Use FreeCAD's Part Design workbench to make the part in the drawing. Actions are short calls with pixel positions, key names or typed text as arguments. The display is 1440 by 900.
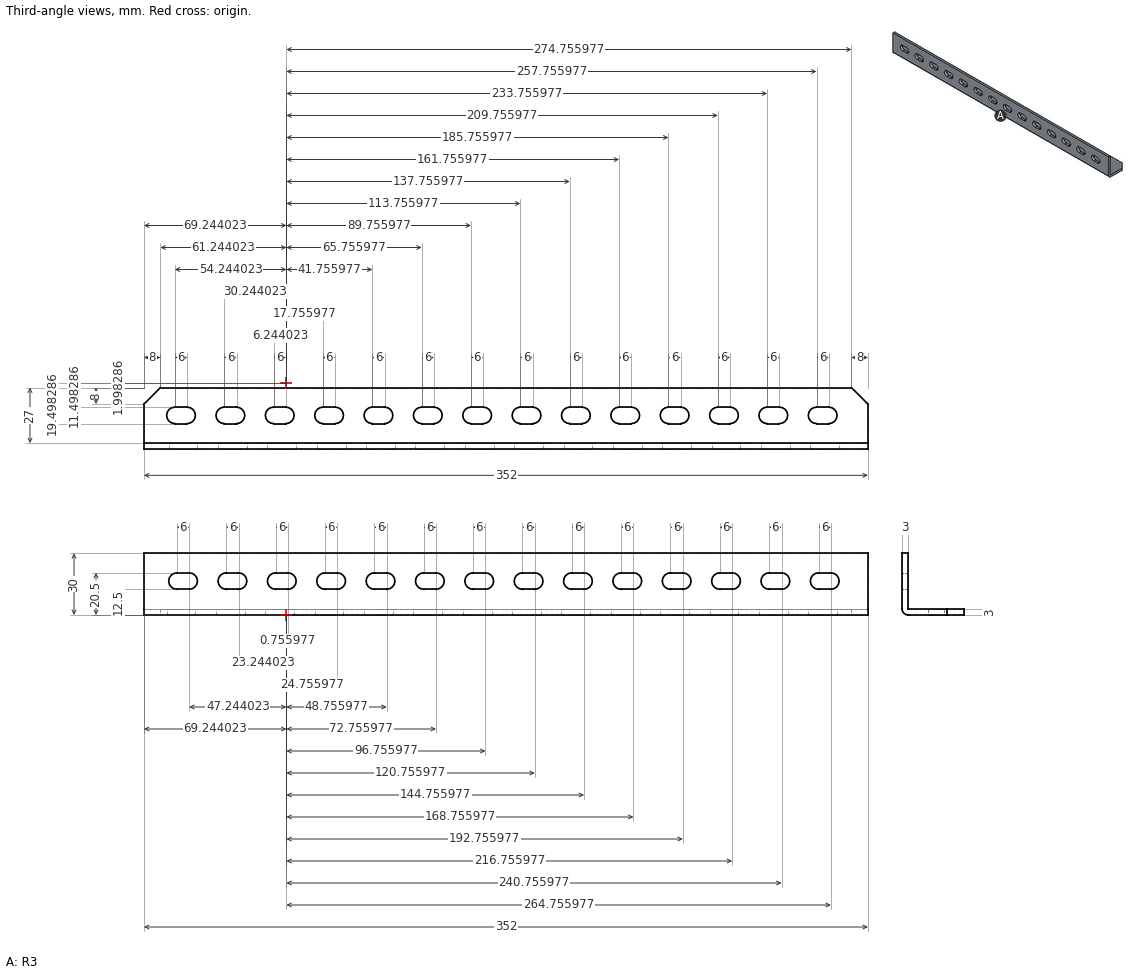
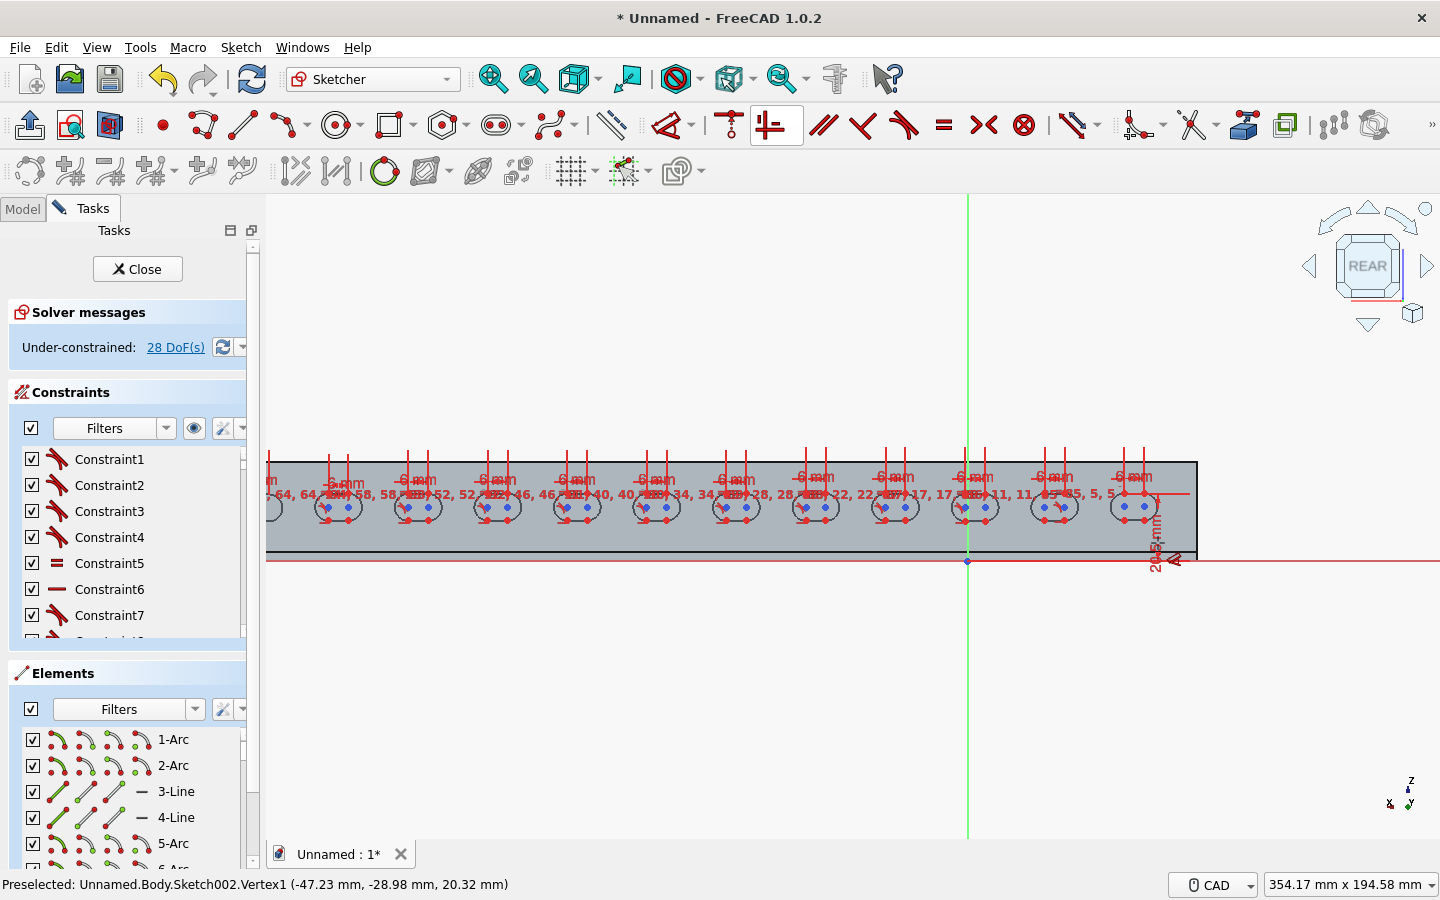
click(1124, 520)
click(934, 541)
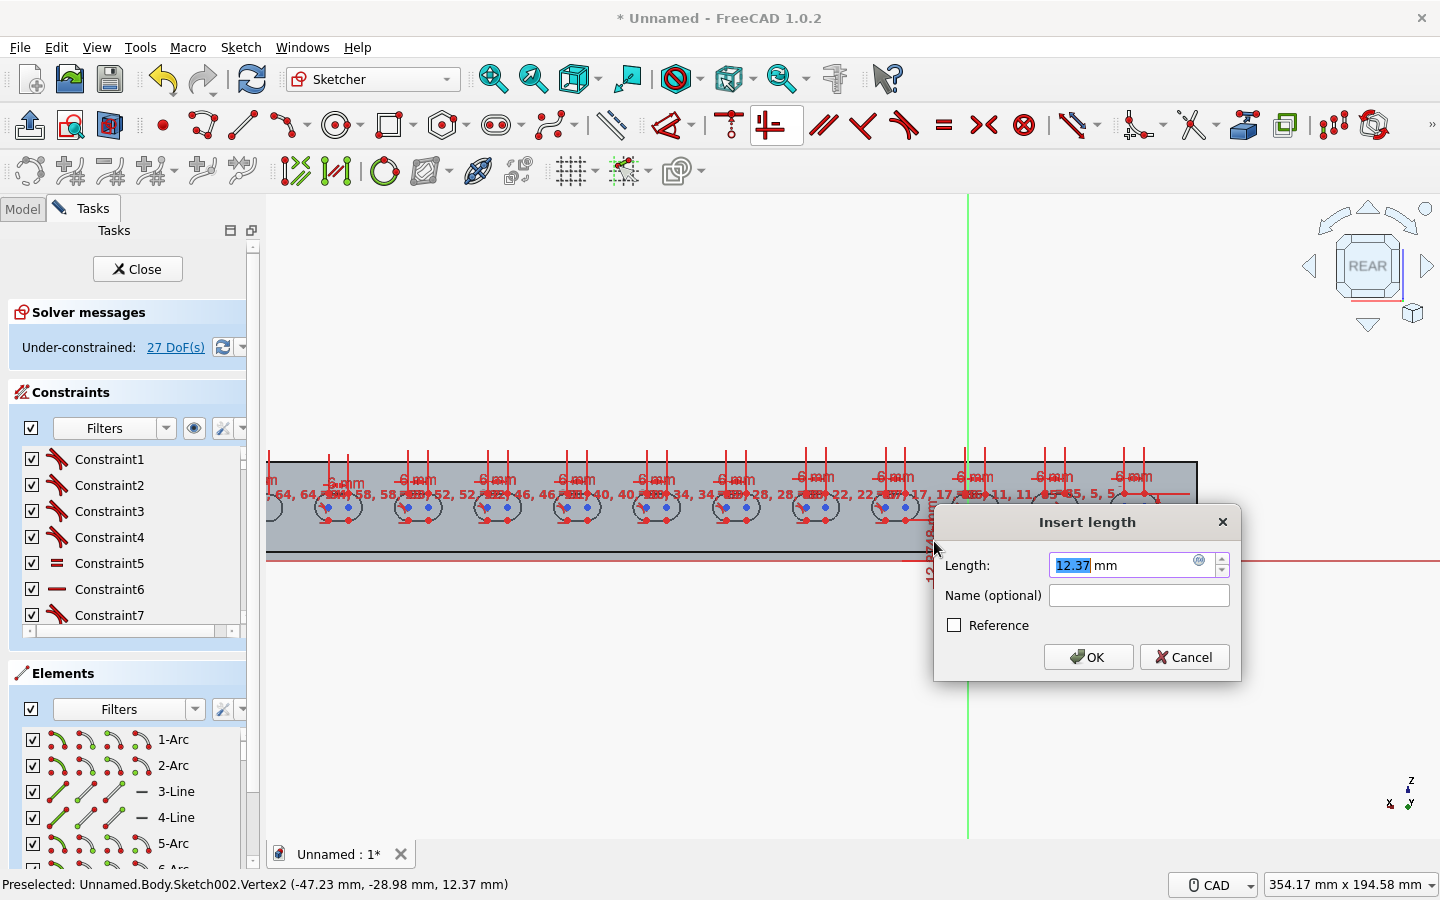
text(12.5)
key(Return)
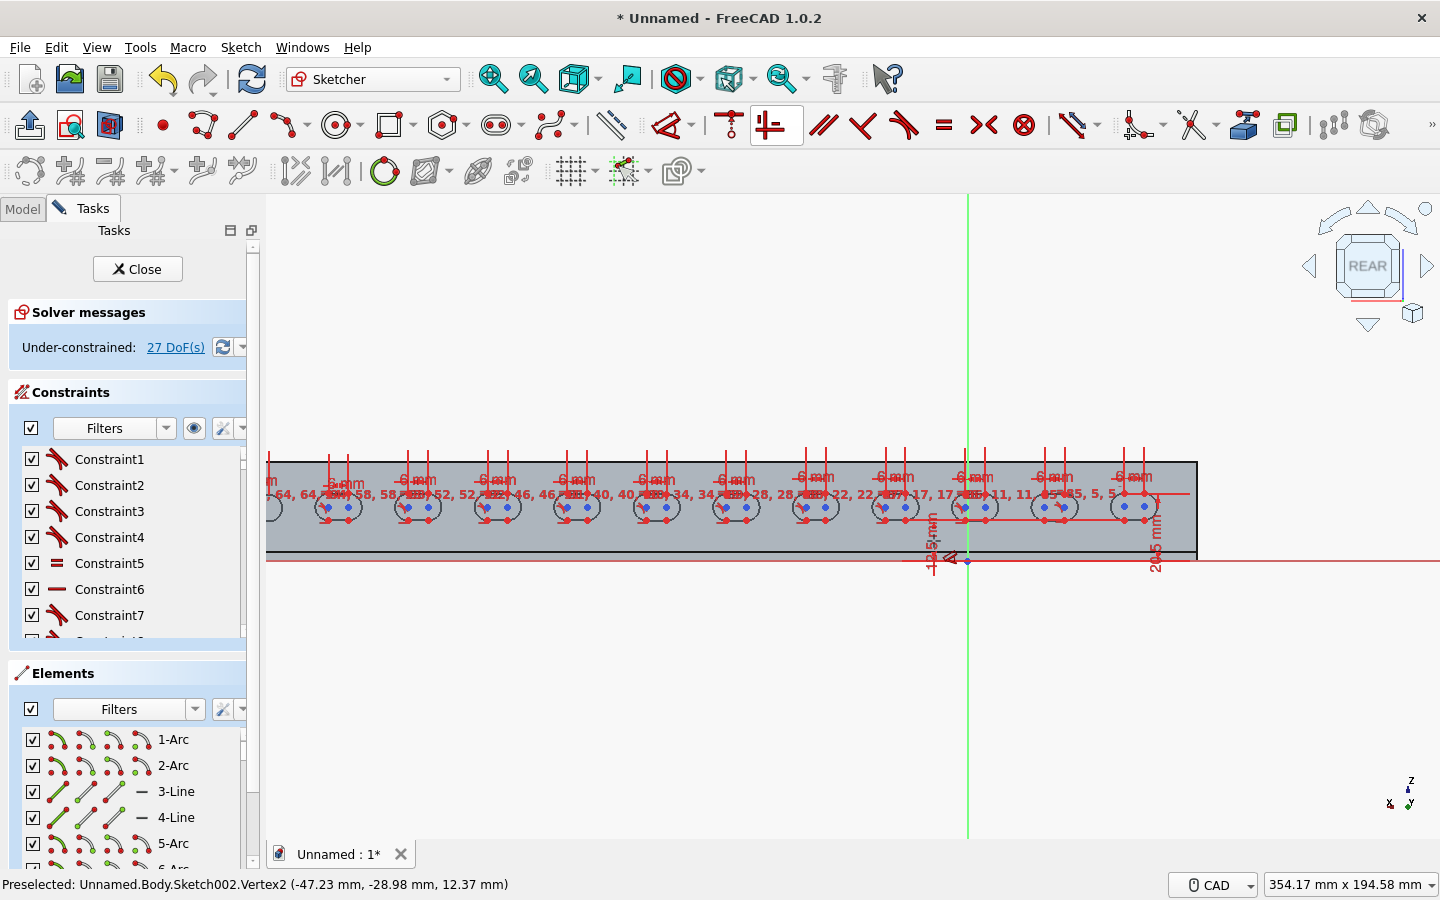
click(1045, 494)
click(1079, 543)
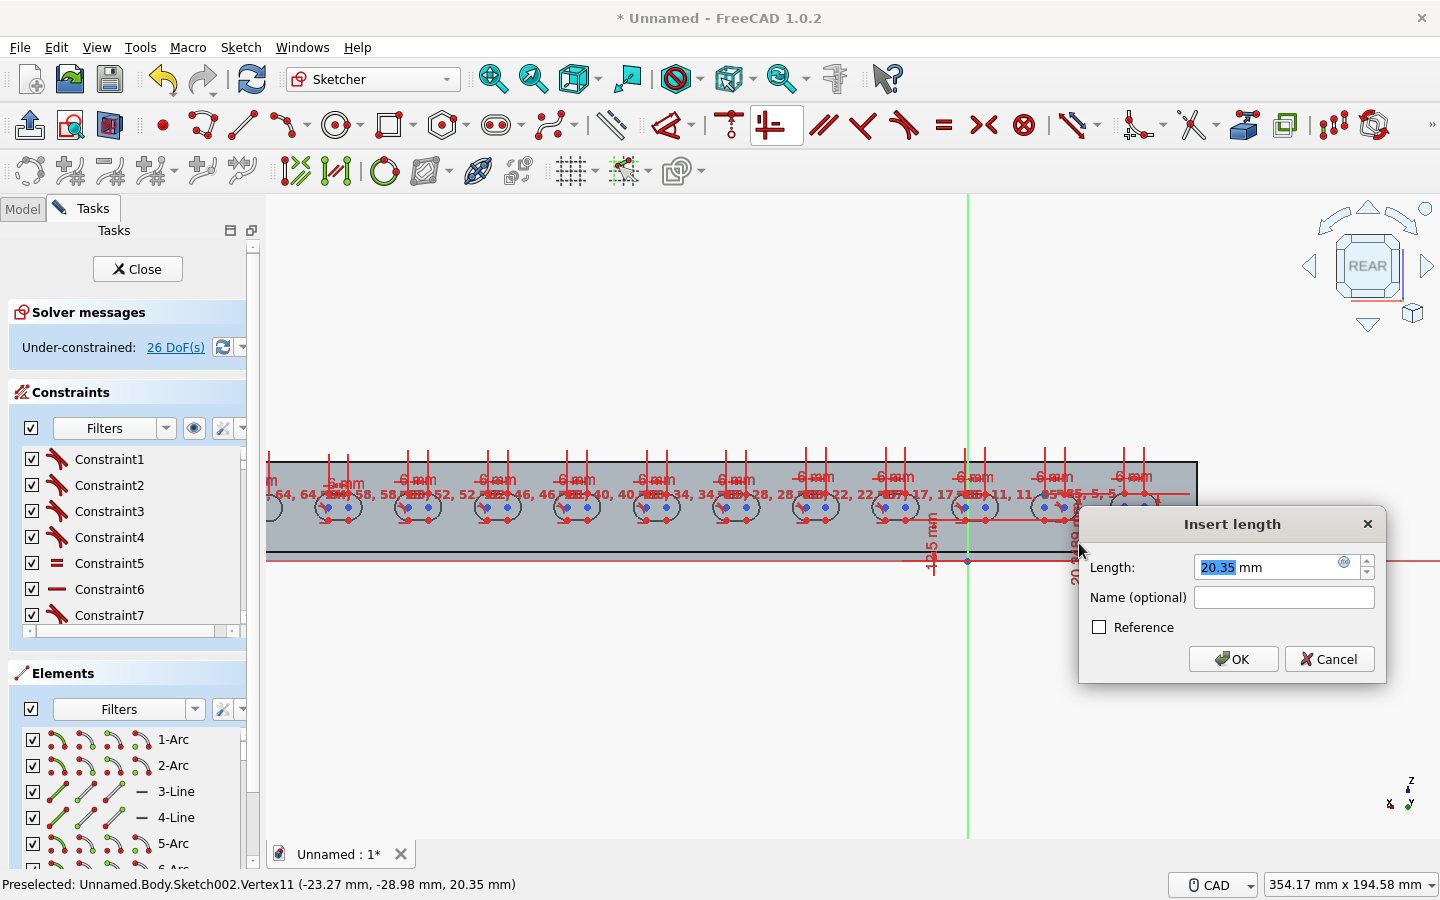
text(20.5)
key(Return)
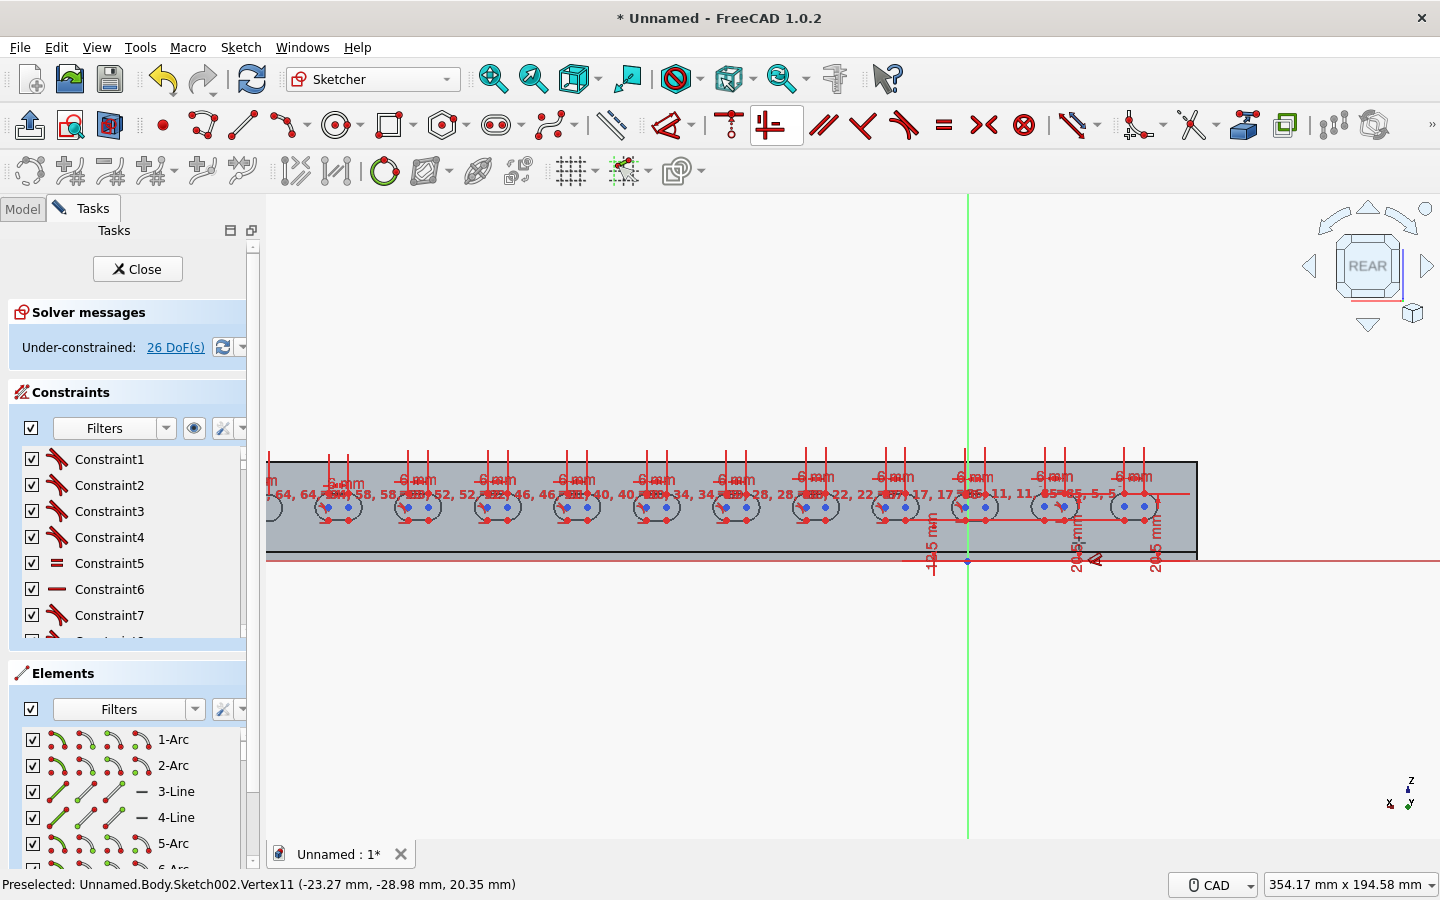
click(965, 494)
click(931, 512)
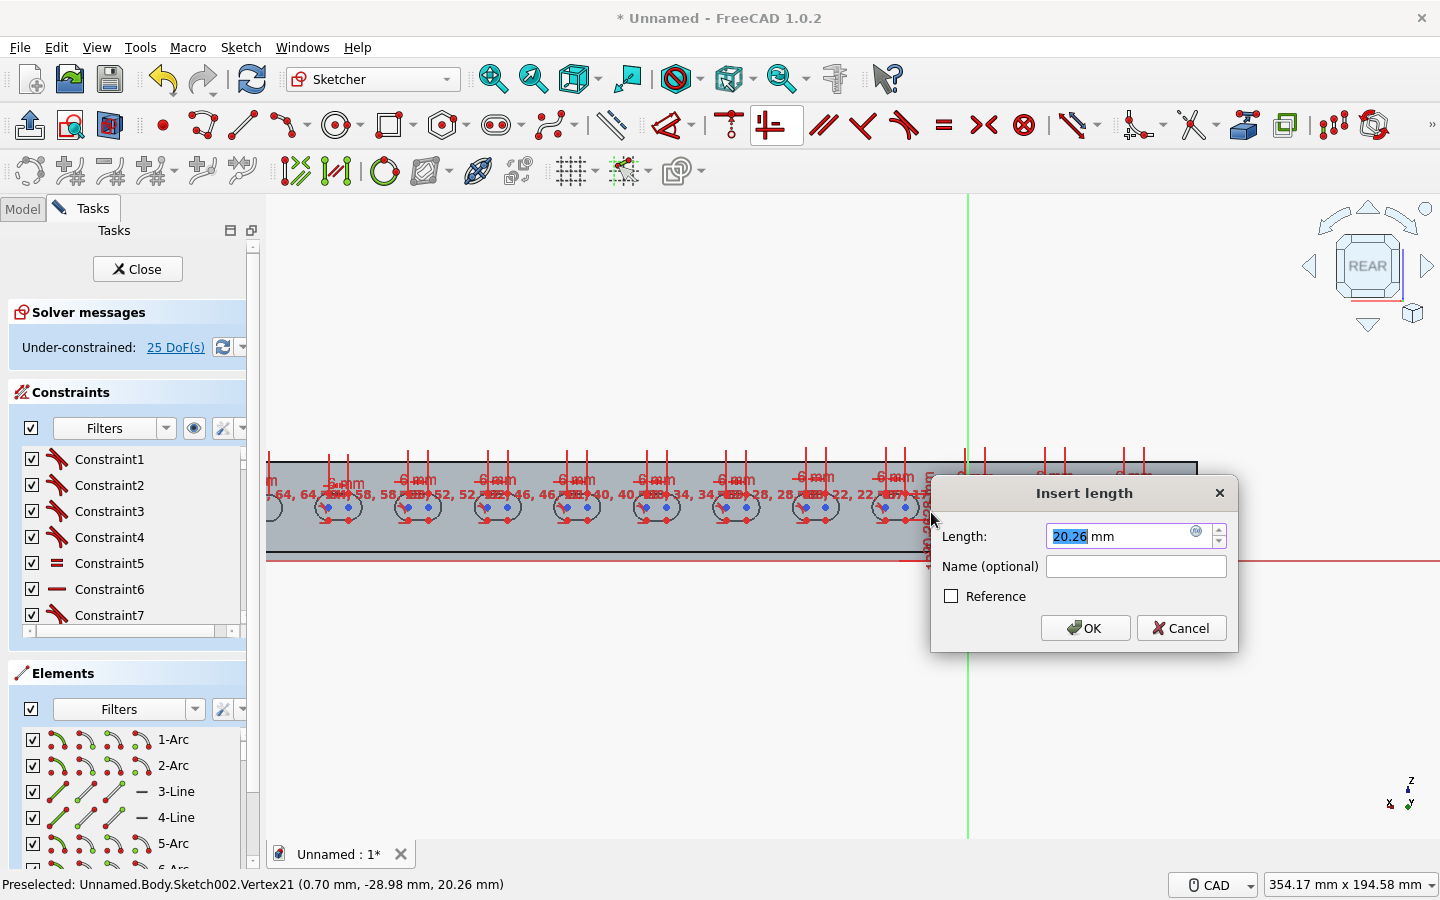
text(20.5)
key(Return)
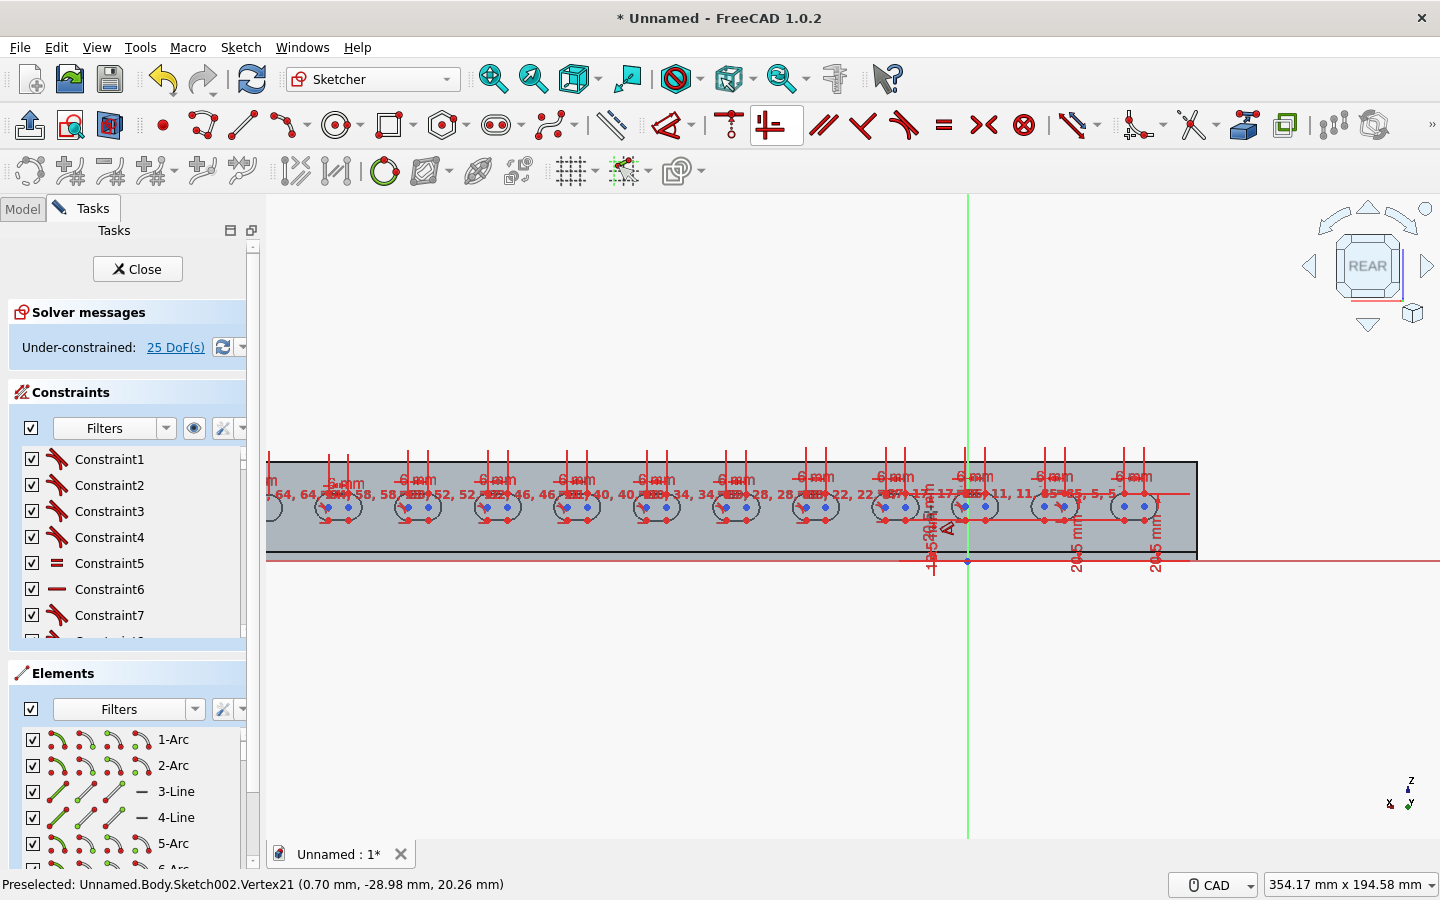
click(886, 494)
click(852, 528)